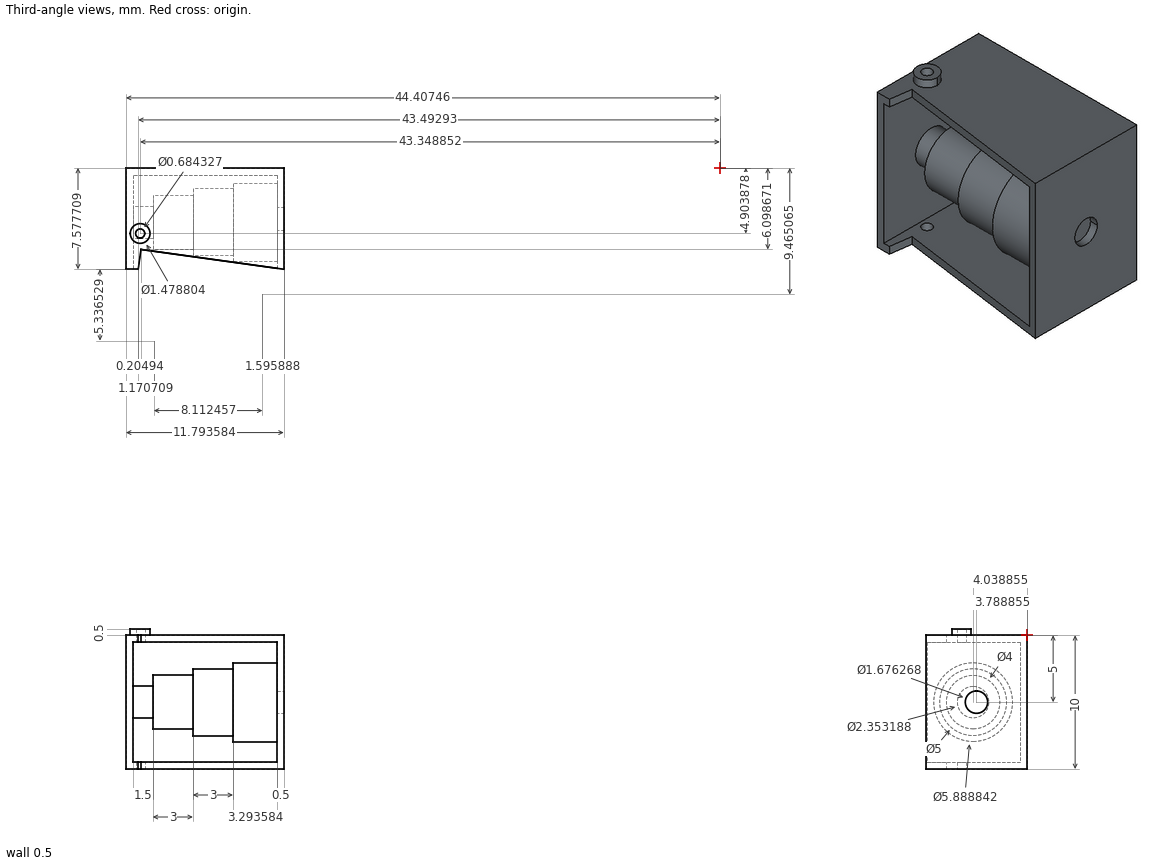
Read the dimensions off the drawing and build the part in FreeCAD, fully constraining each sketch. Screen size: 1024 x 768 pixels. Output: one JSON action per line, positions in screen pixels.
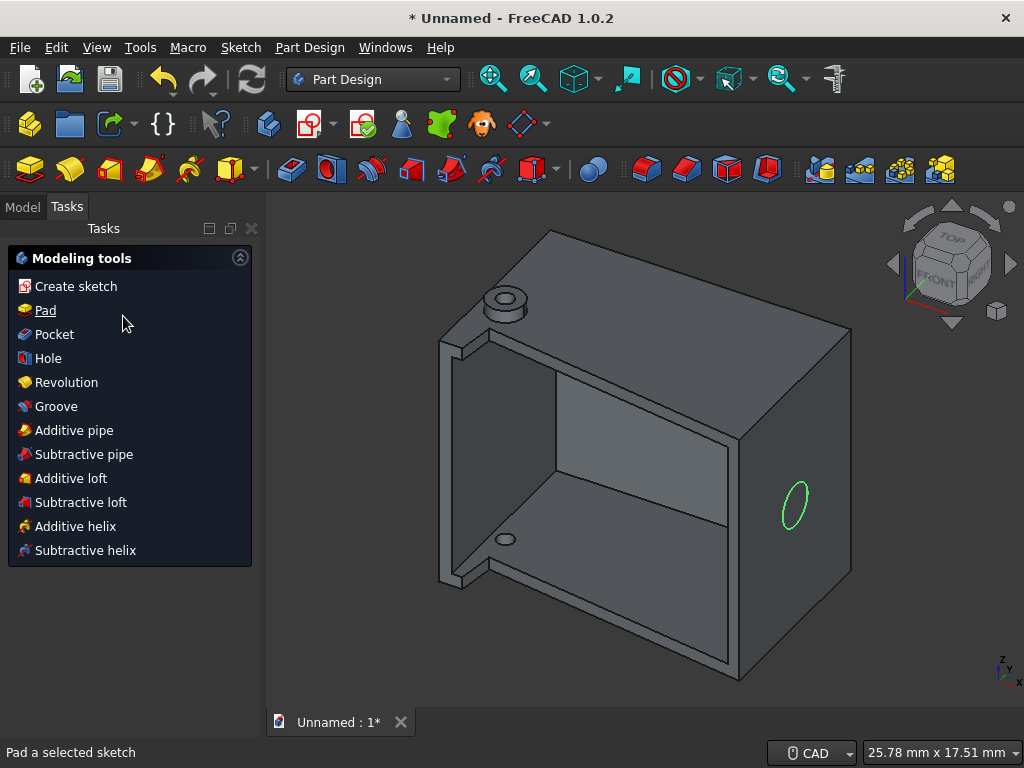
{"action": "left_click", "coordinate": [292, 170]}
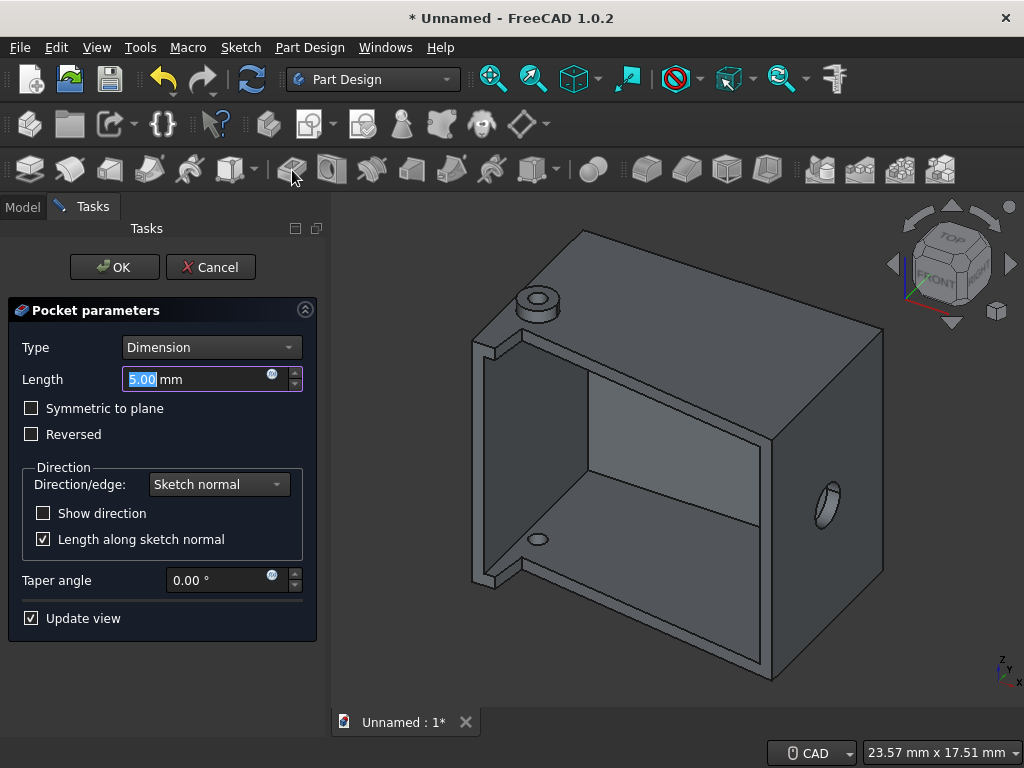
{"action": "left_click", "coordinate": [212, 348]}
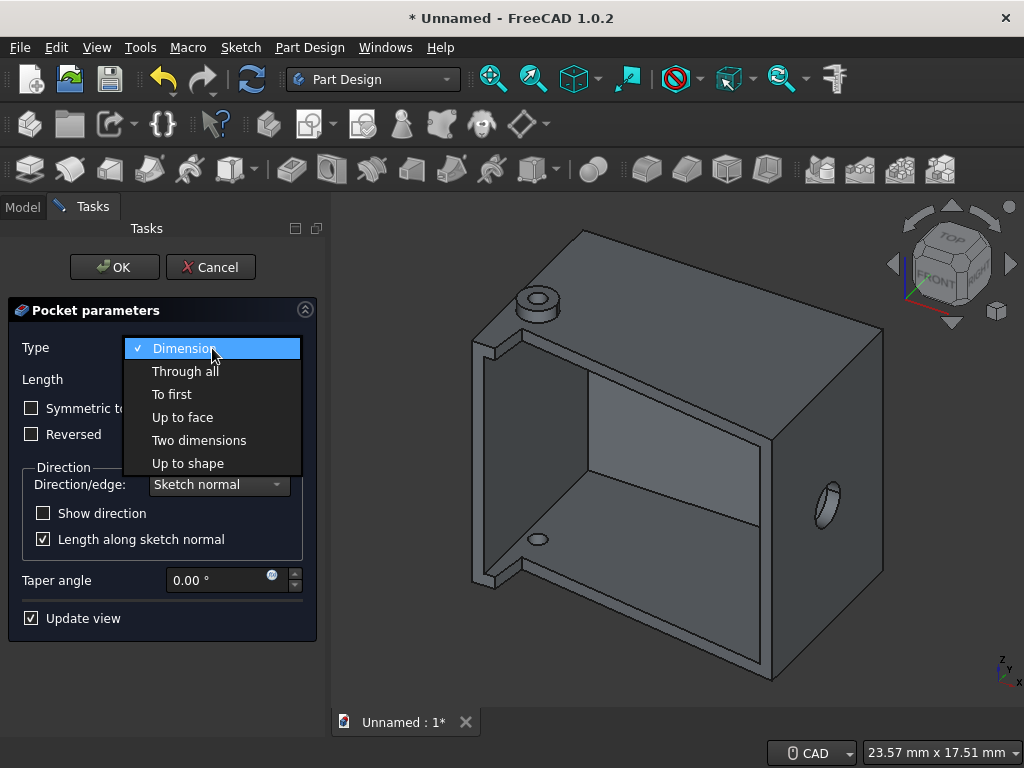
{"action": "left_click", "coordinate": [212, 440]}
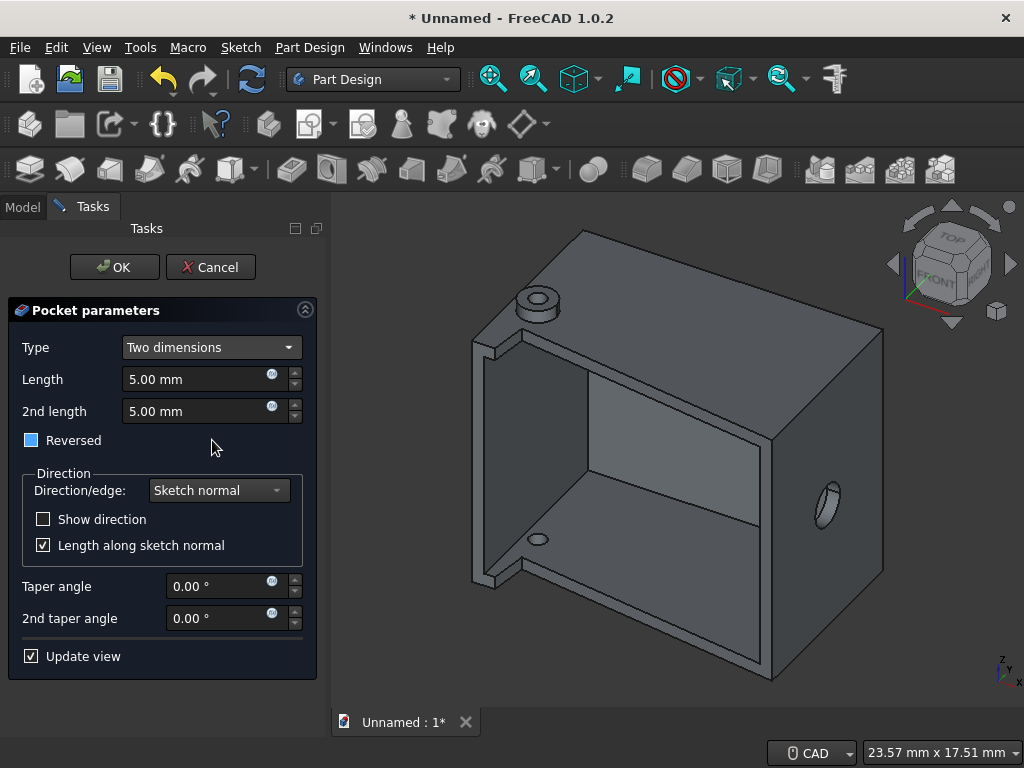
{"action": "triple_click", "coordinate": [204, 379]}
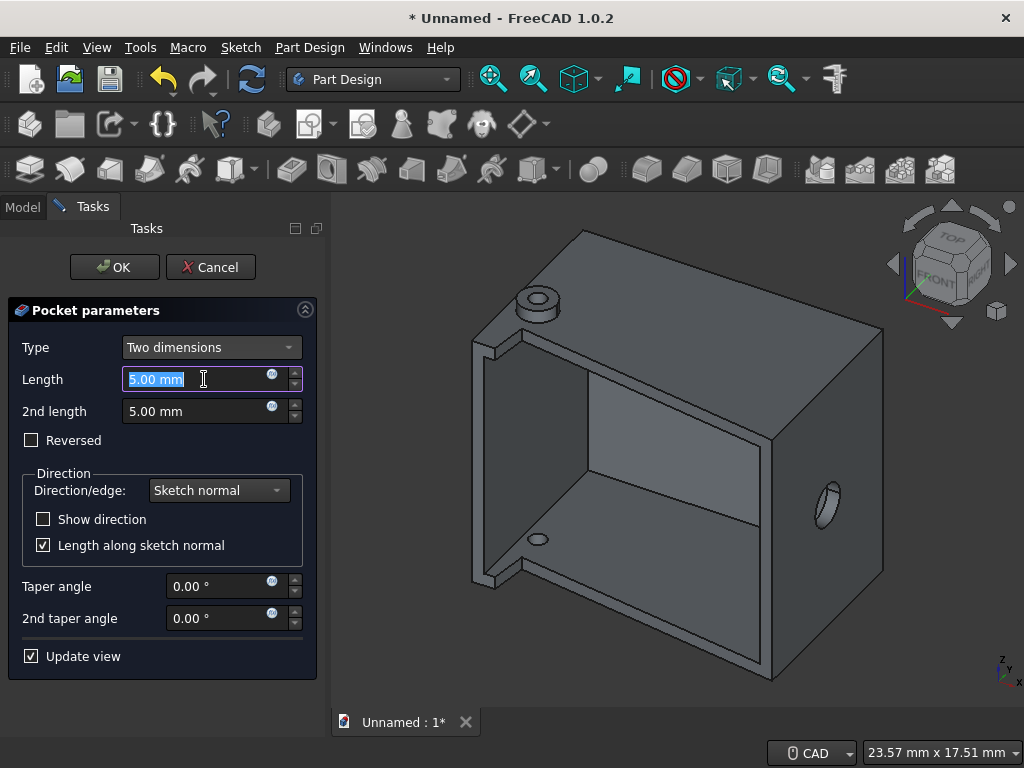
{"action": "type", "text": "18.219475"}
{"action": "key", "text": "Tab"}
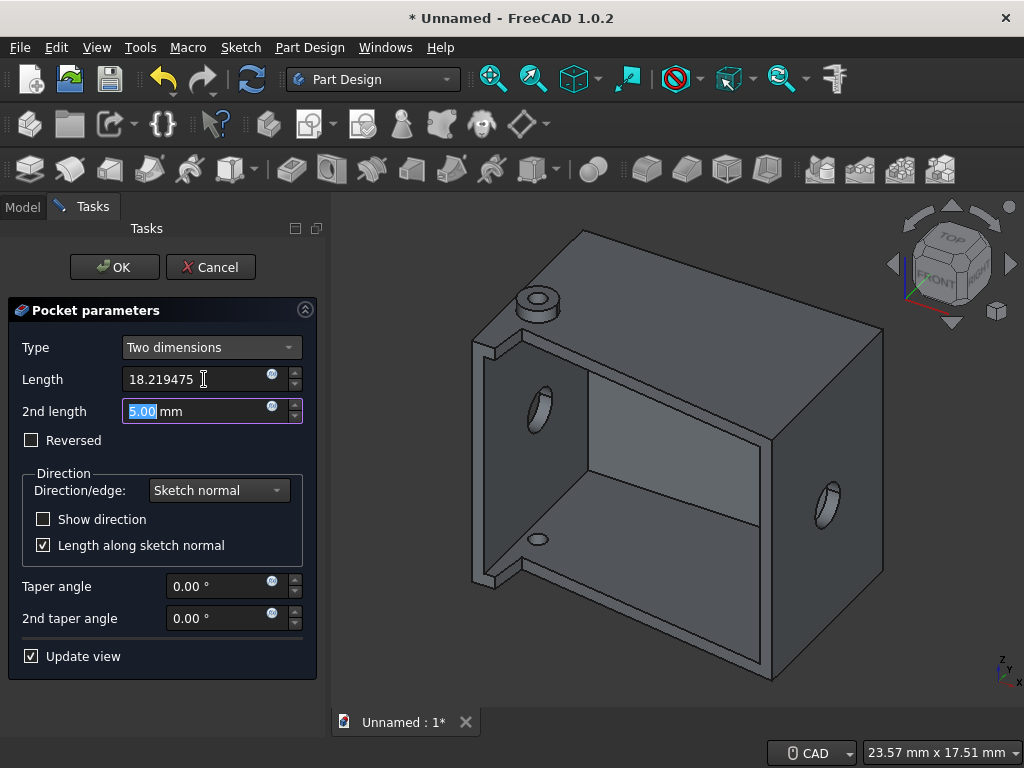
{"action": "type", "text": "0.5"}
{"action": "key", "text": "Tab"}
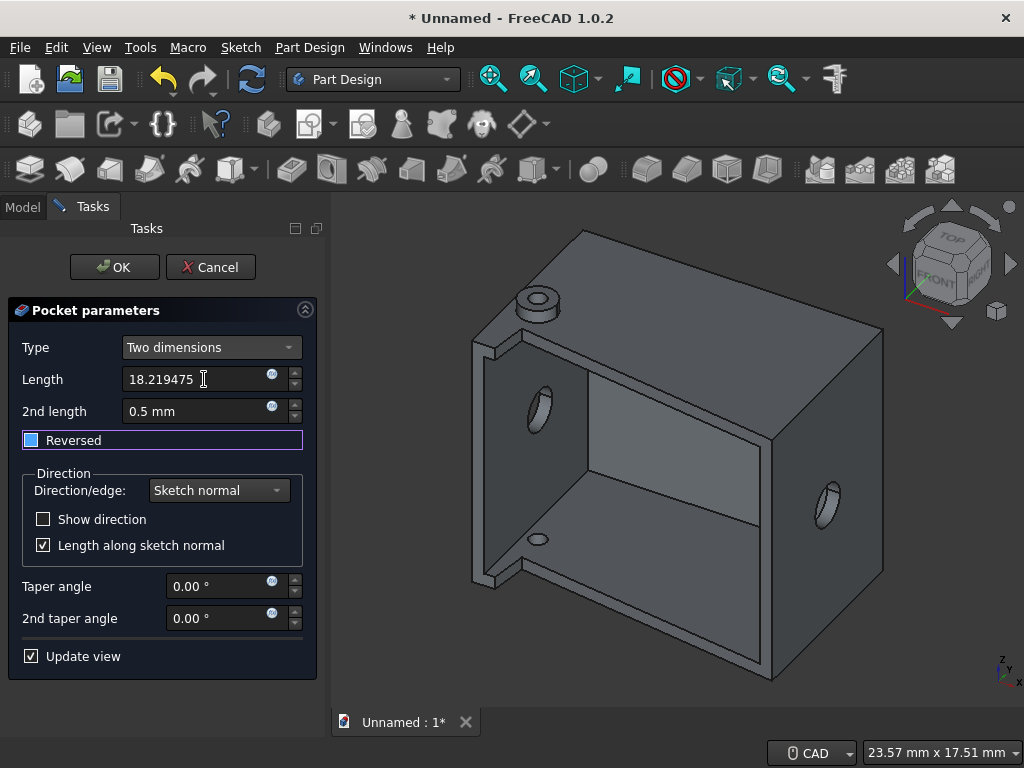
{"action": "left_click", "coordinate": [30, 440]}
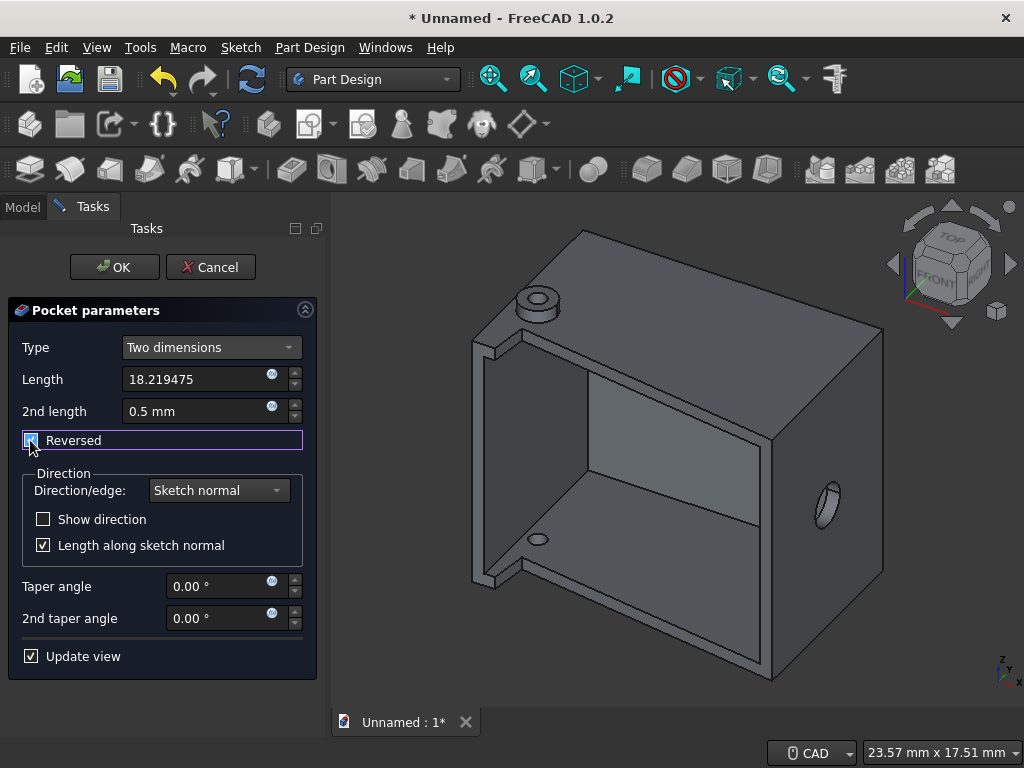
{"action": "left_click", "coordinate": [115, 267]}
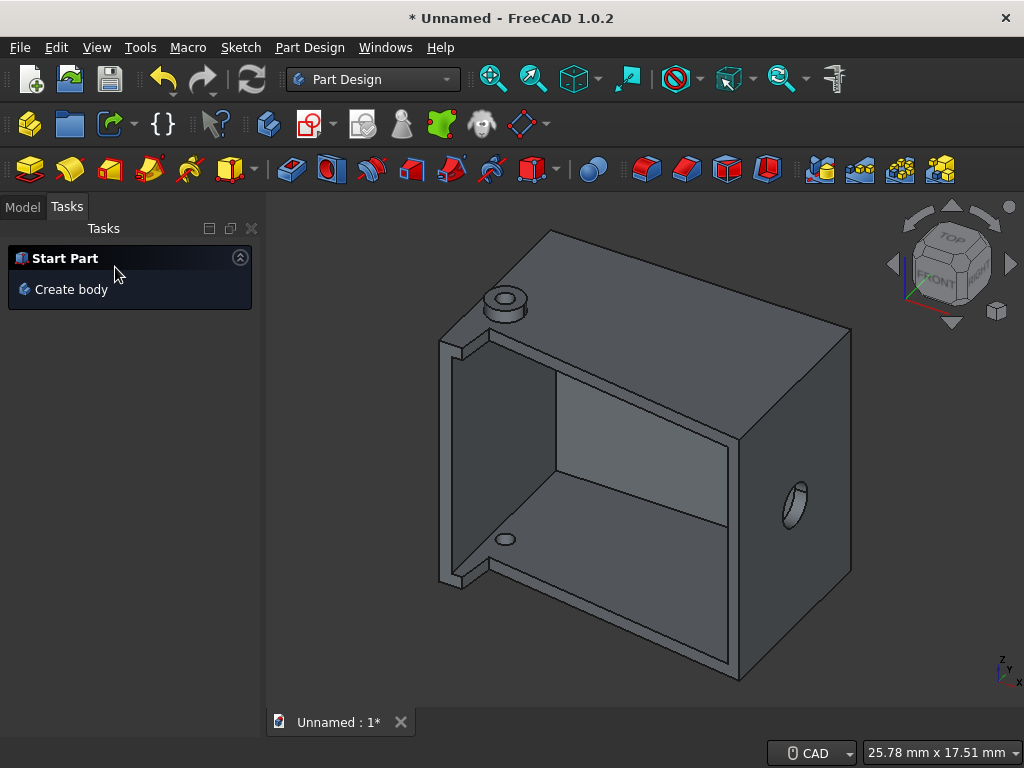
{"action": "left_click", "coordinate": [504, 413]}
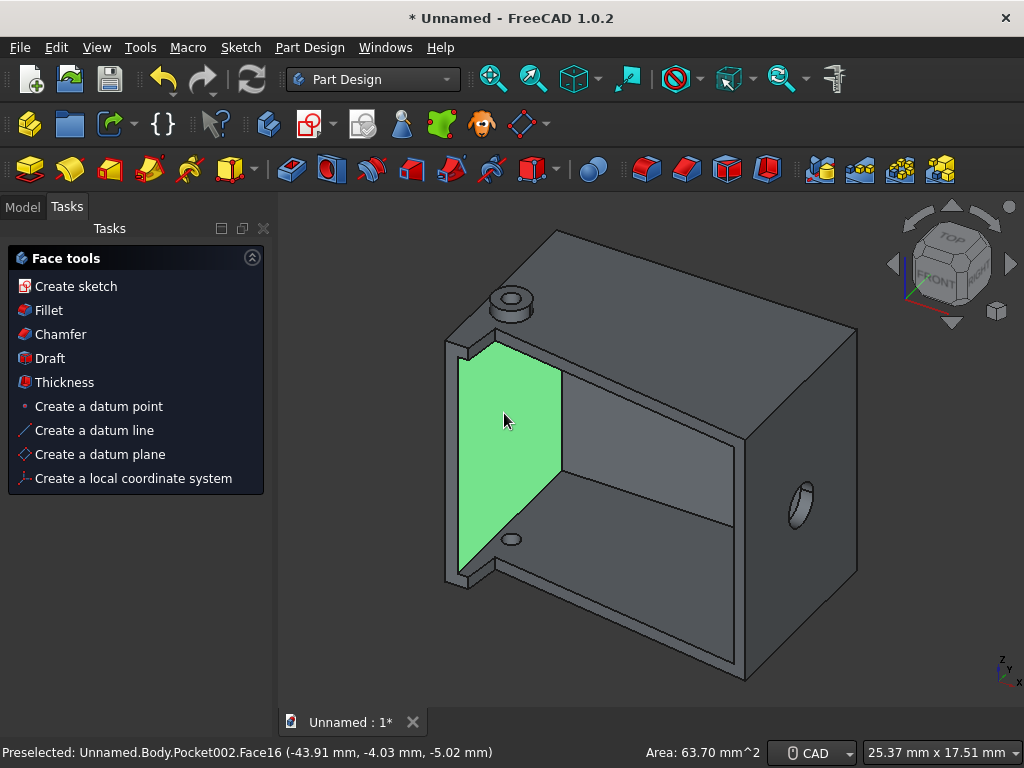
{"action": "left_click", "coordinate": [310, 124]}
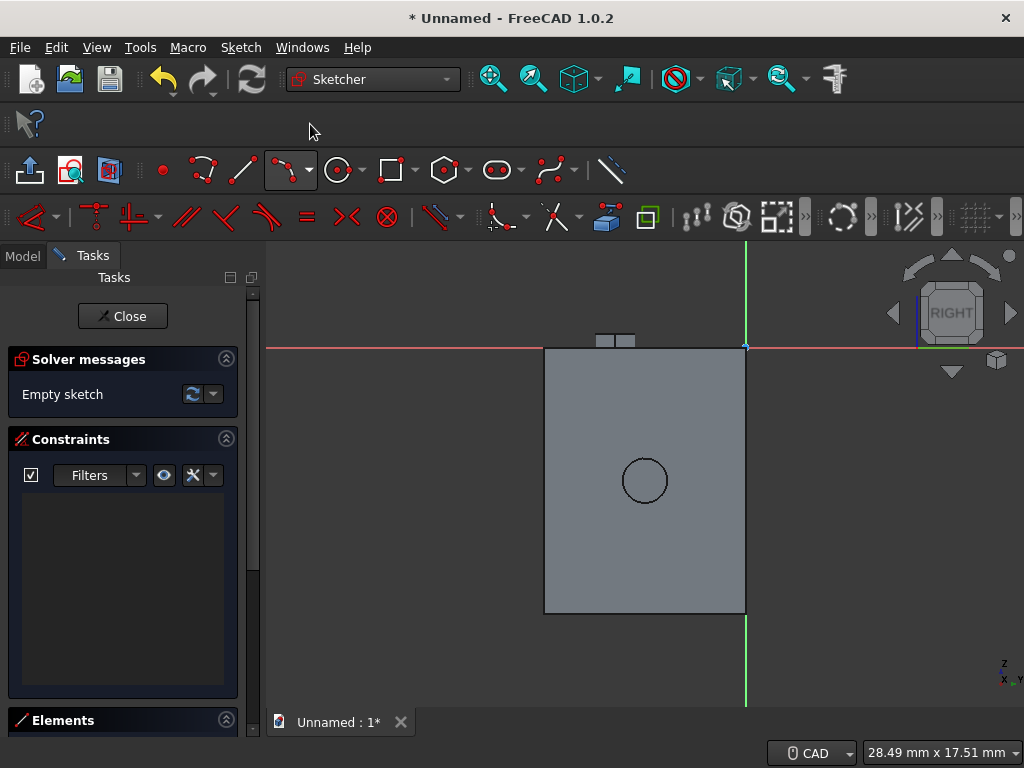
{"action": "scroll", "coordinate": [654, 482], "scroll_direction": "up", "scroll_amount": 8}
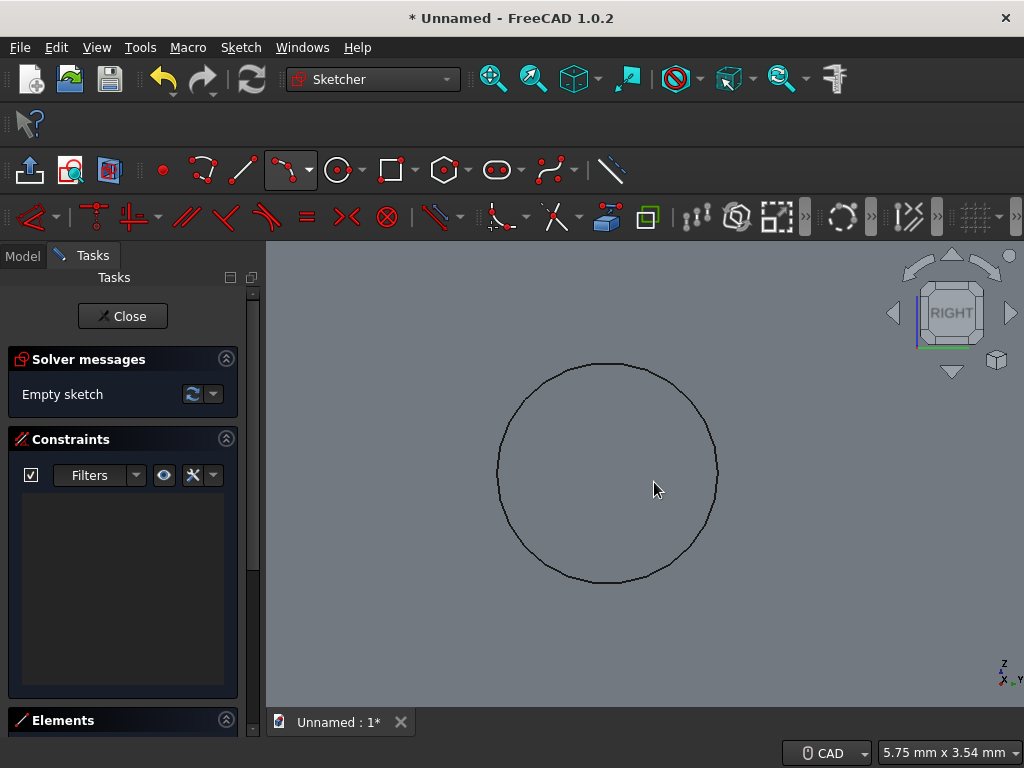
{"action": "left_click", "coordinate": [338, 170]}